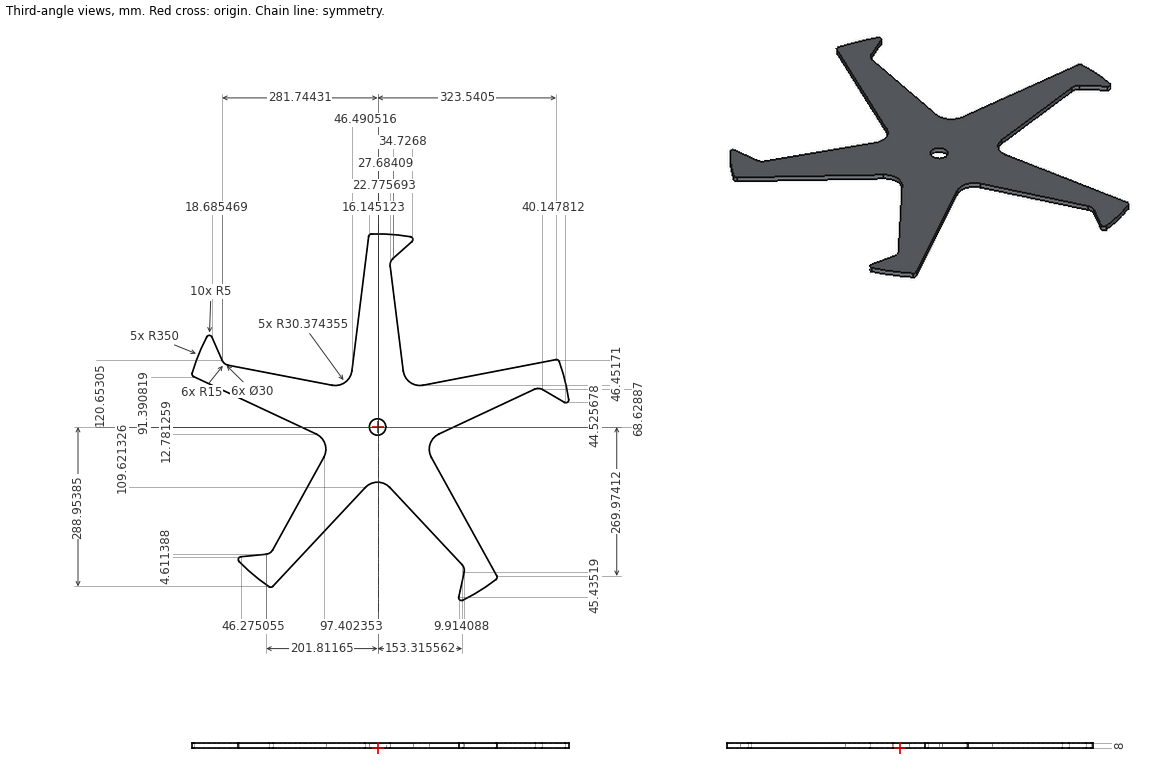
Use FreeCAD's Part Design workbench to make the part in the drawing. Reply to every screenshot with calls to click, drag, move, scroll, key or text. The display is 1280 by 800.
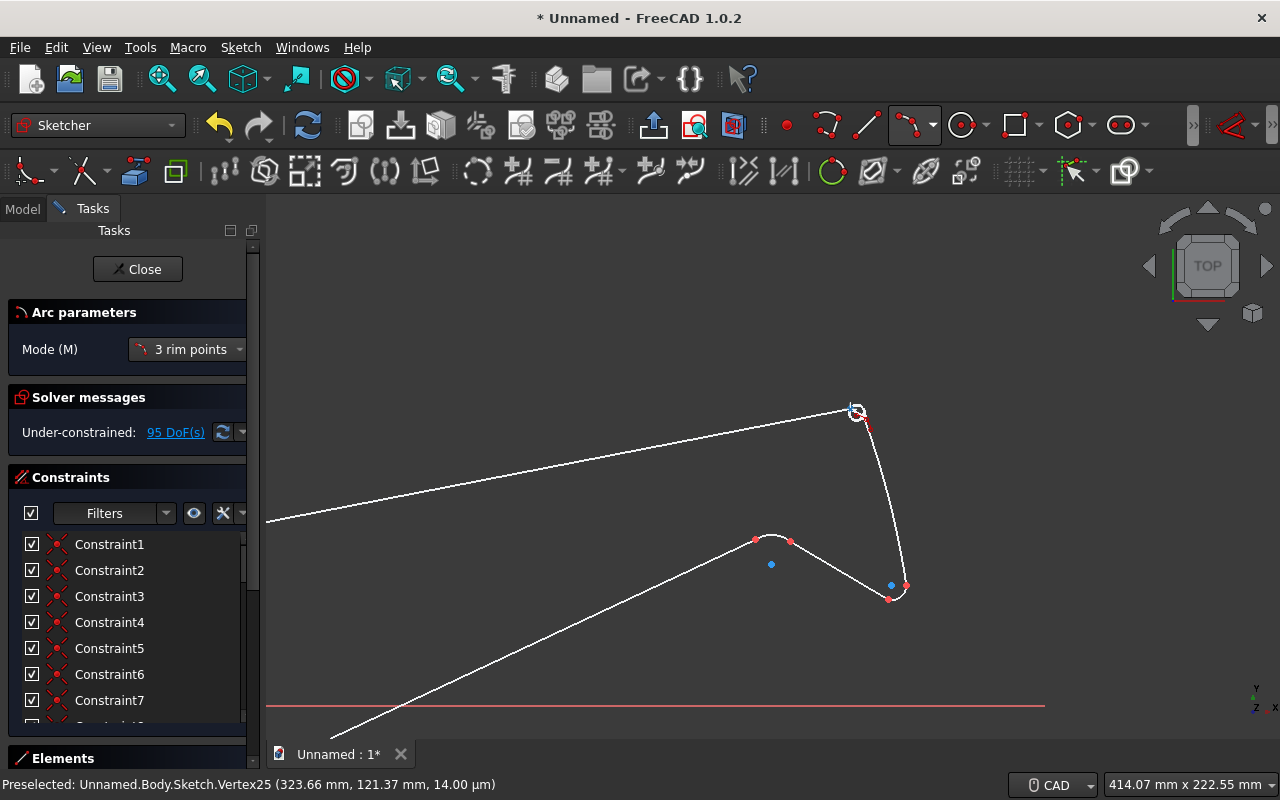
scroll(858, 409, up, 9)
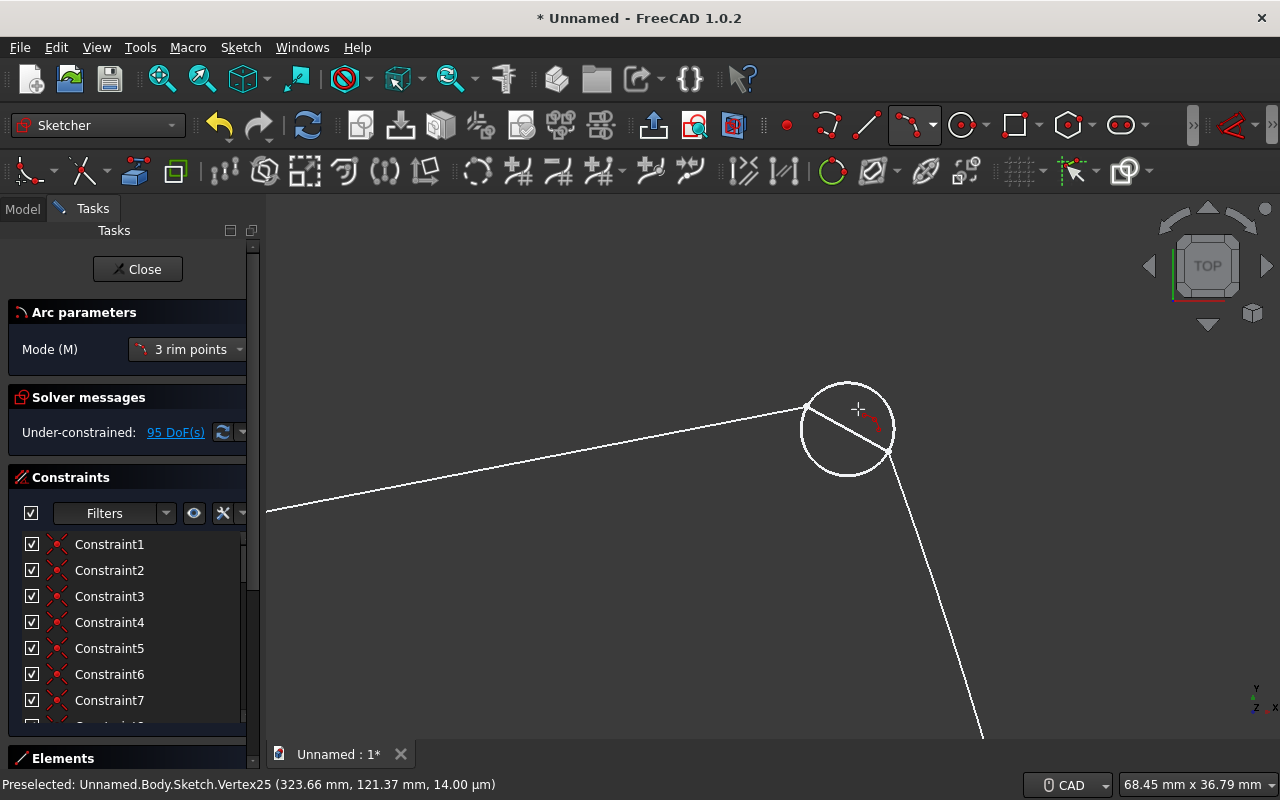
click(856, 404)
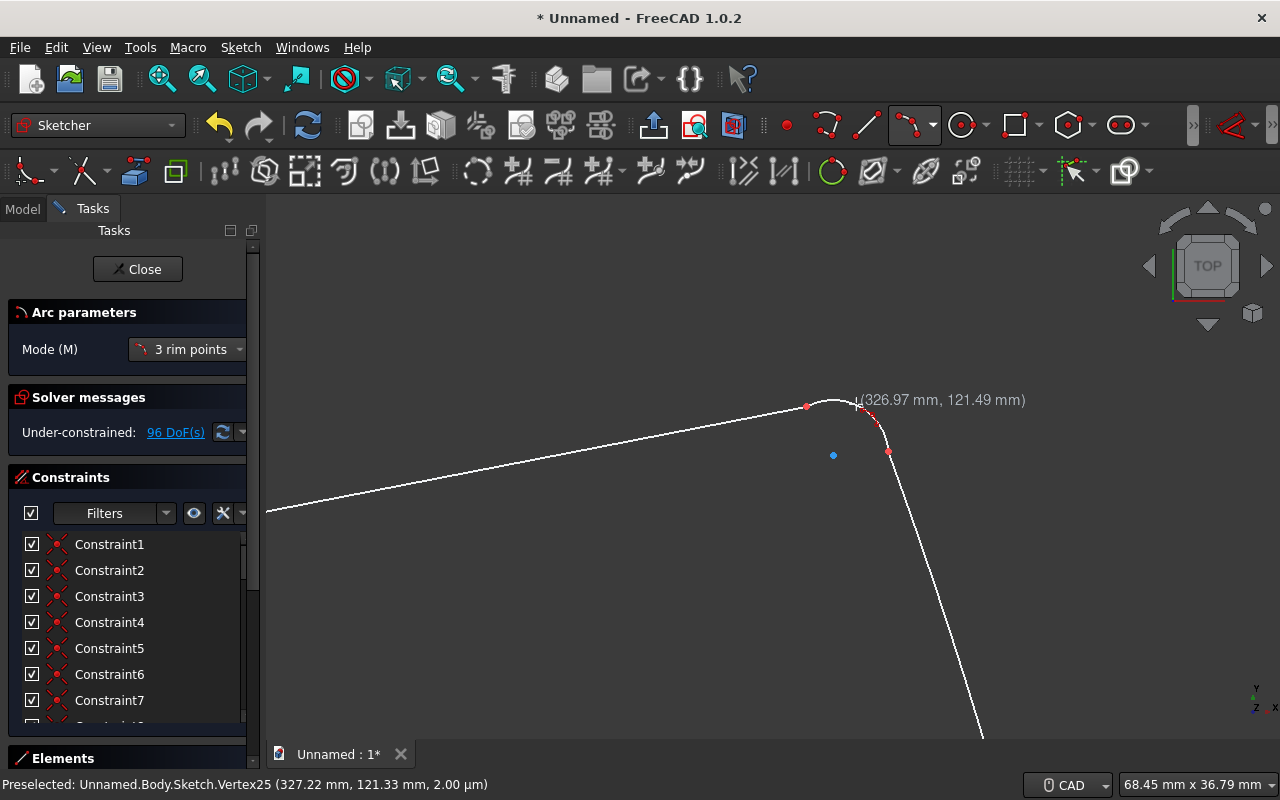
scroll(901, 404, down, 16)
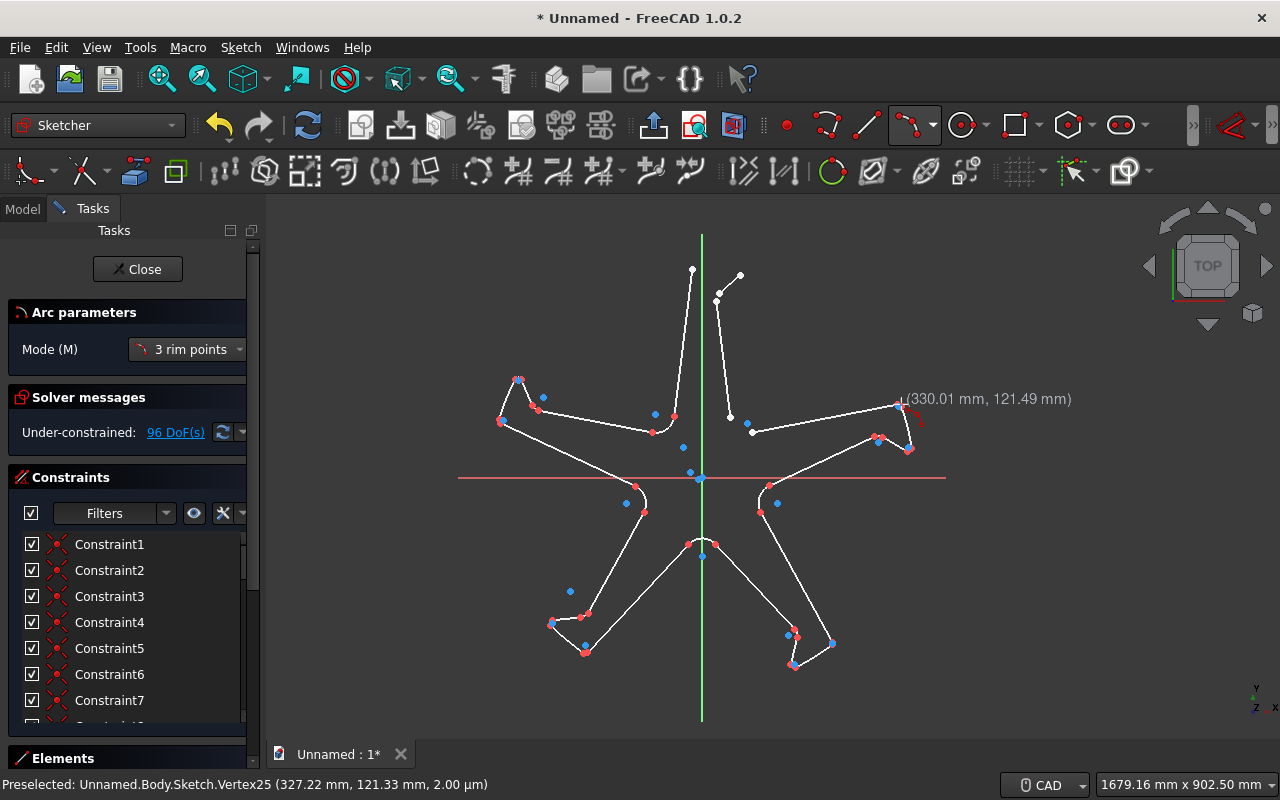
click(752, 433)
click(730, 417)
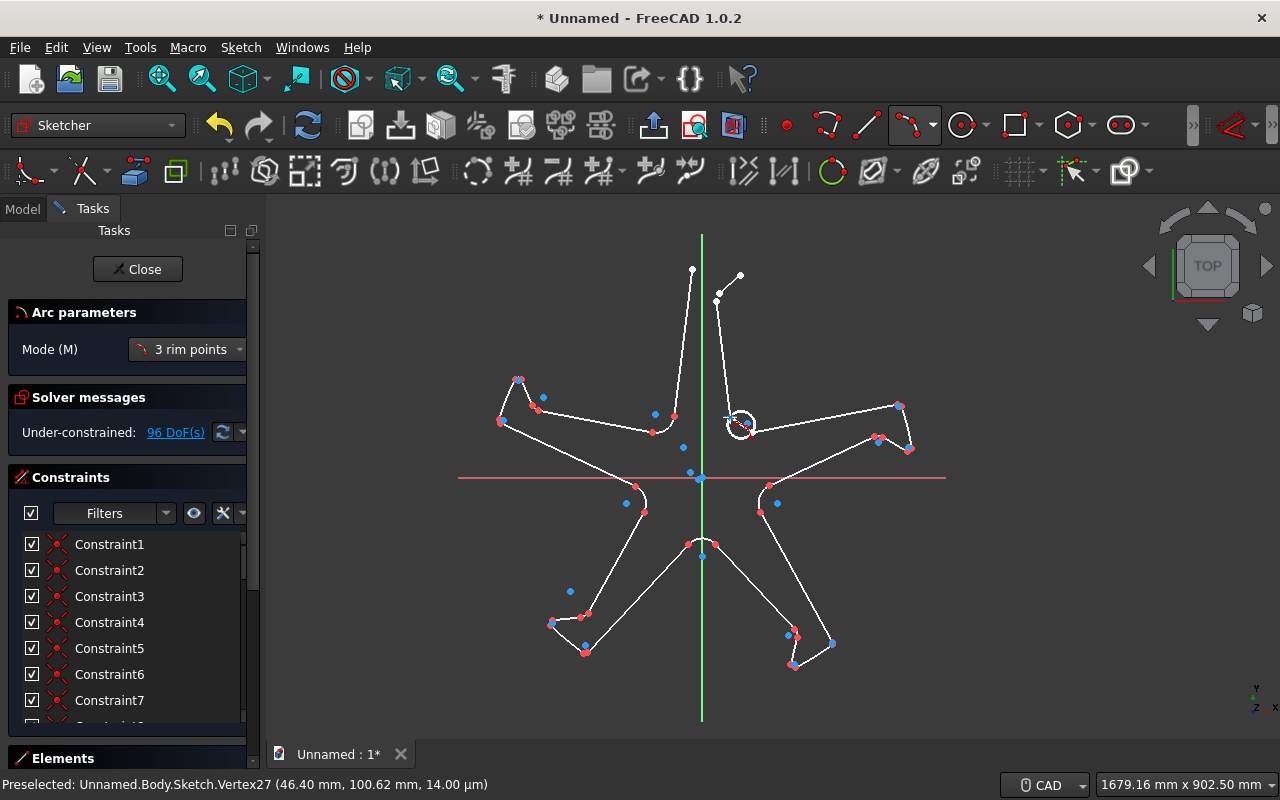
scroll(738, 429, up, 6)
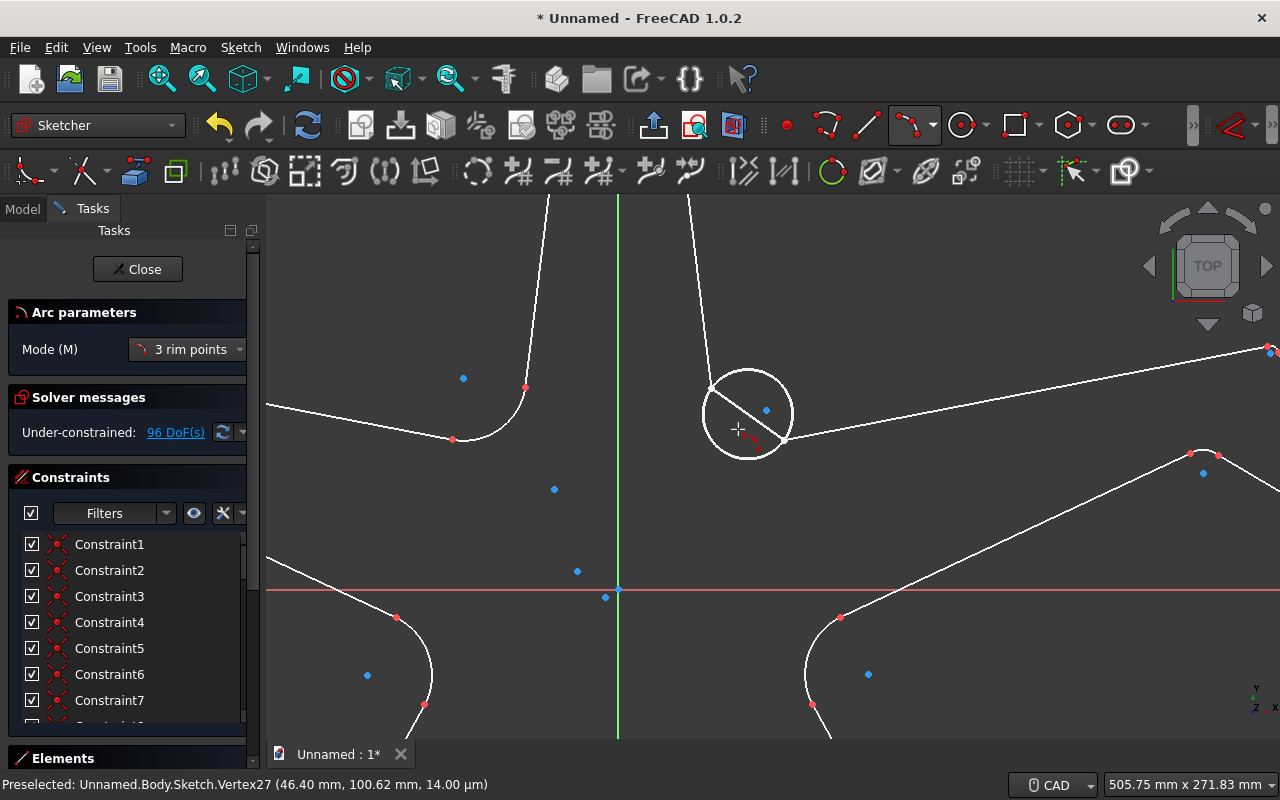
click(736, 428)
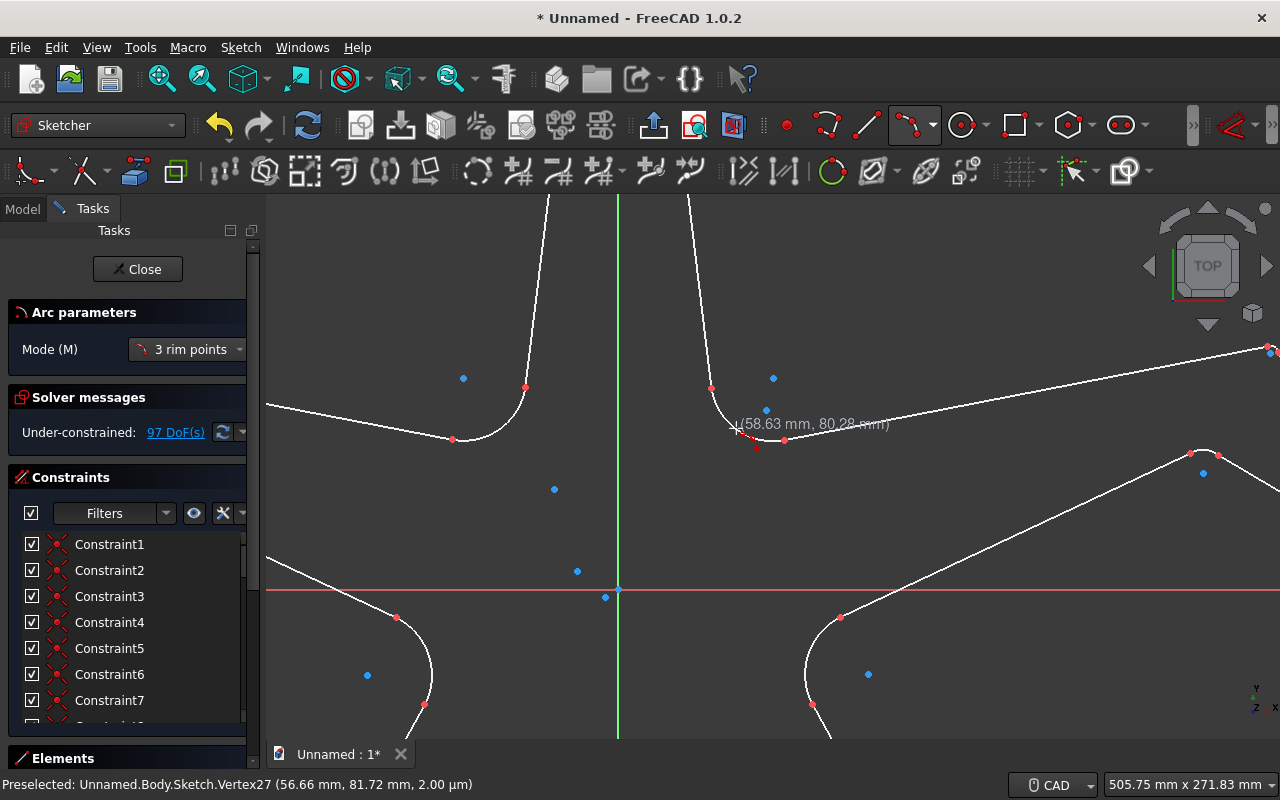
scroll(729, 438, down, 7)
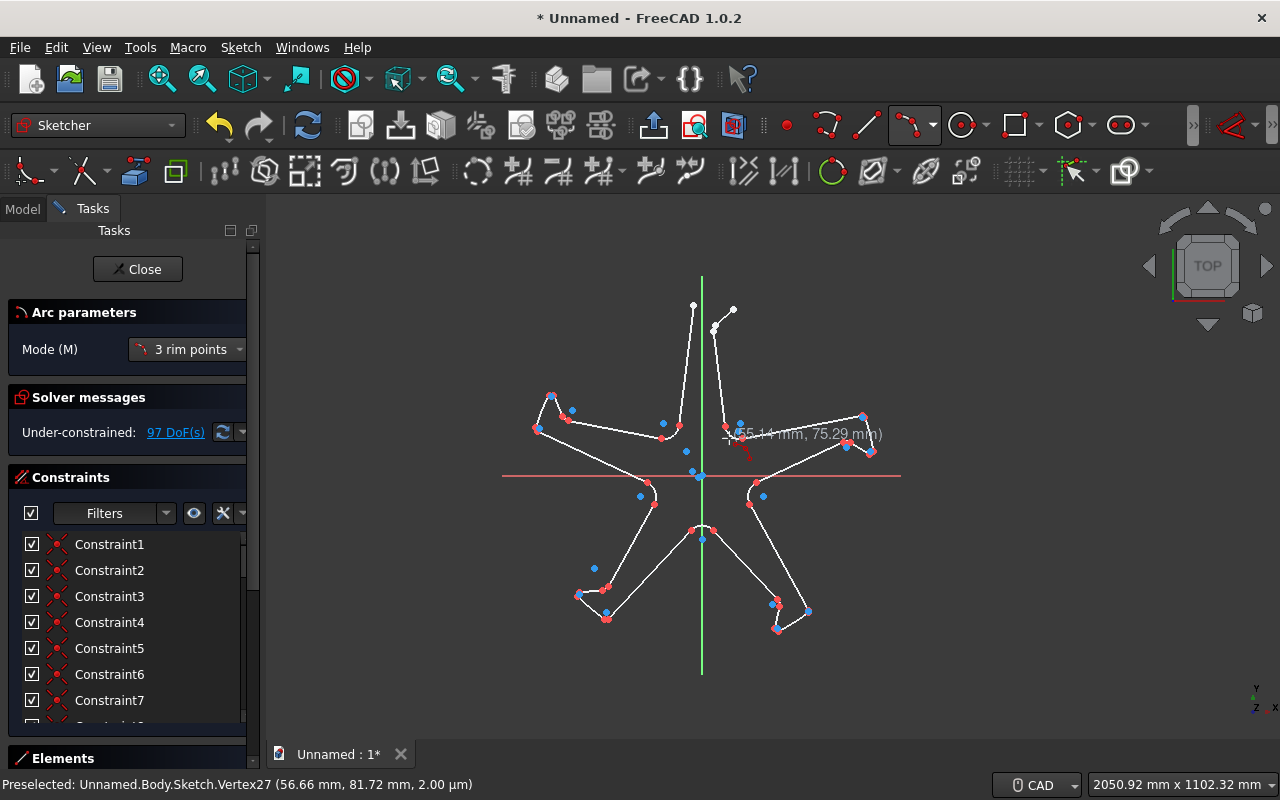
scroll(713, 331, up, 5)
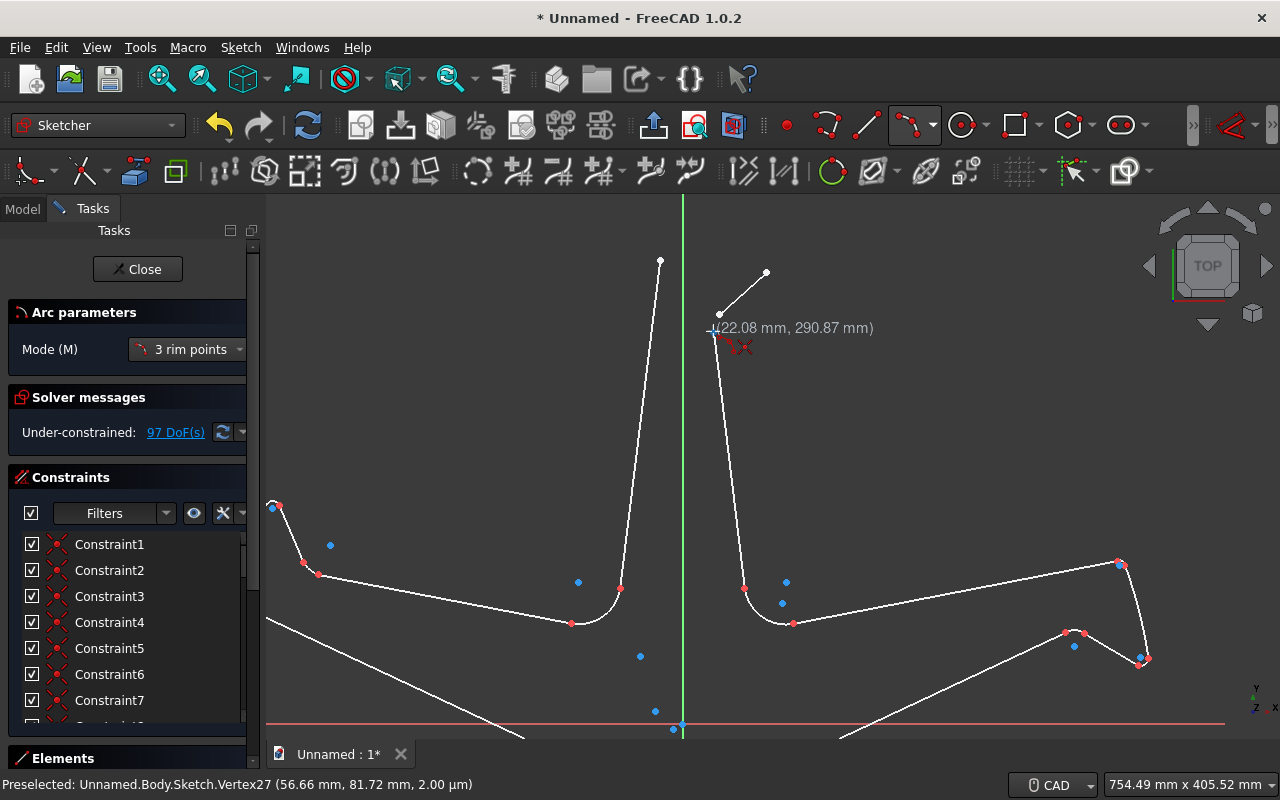
click(714, 333)
click(720, 315)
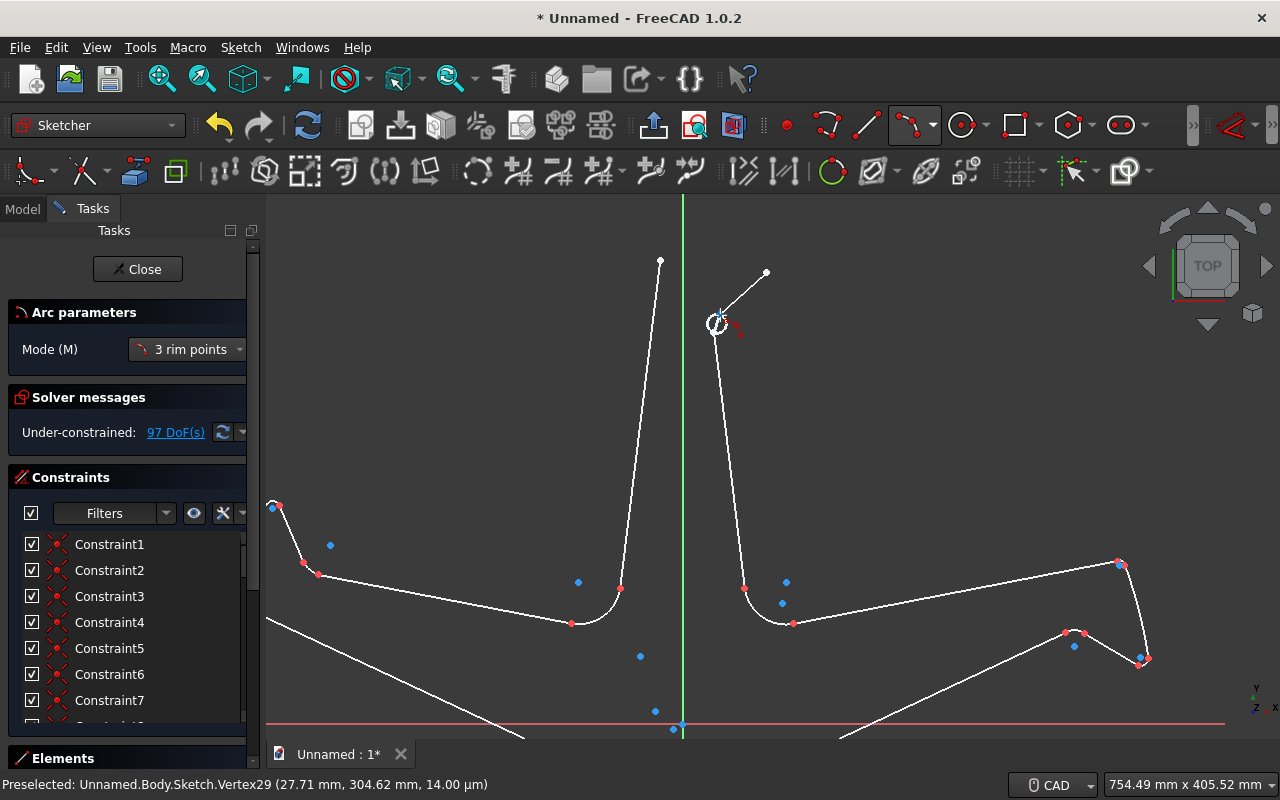
scroll(714, 322, up, 10)